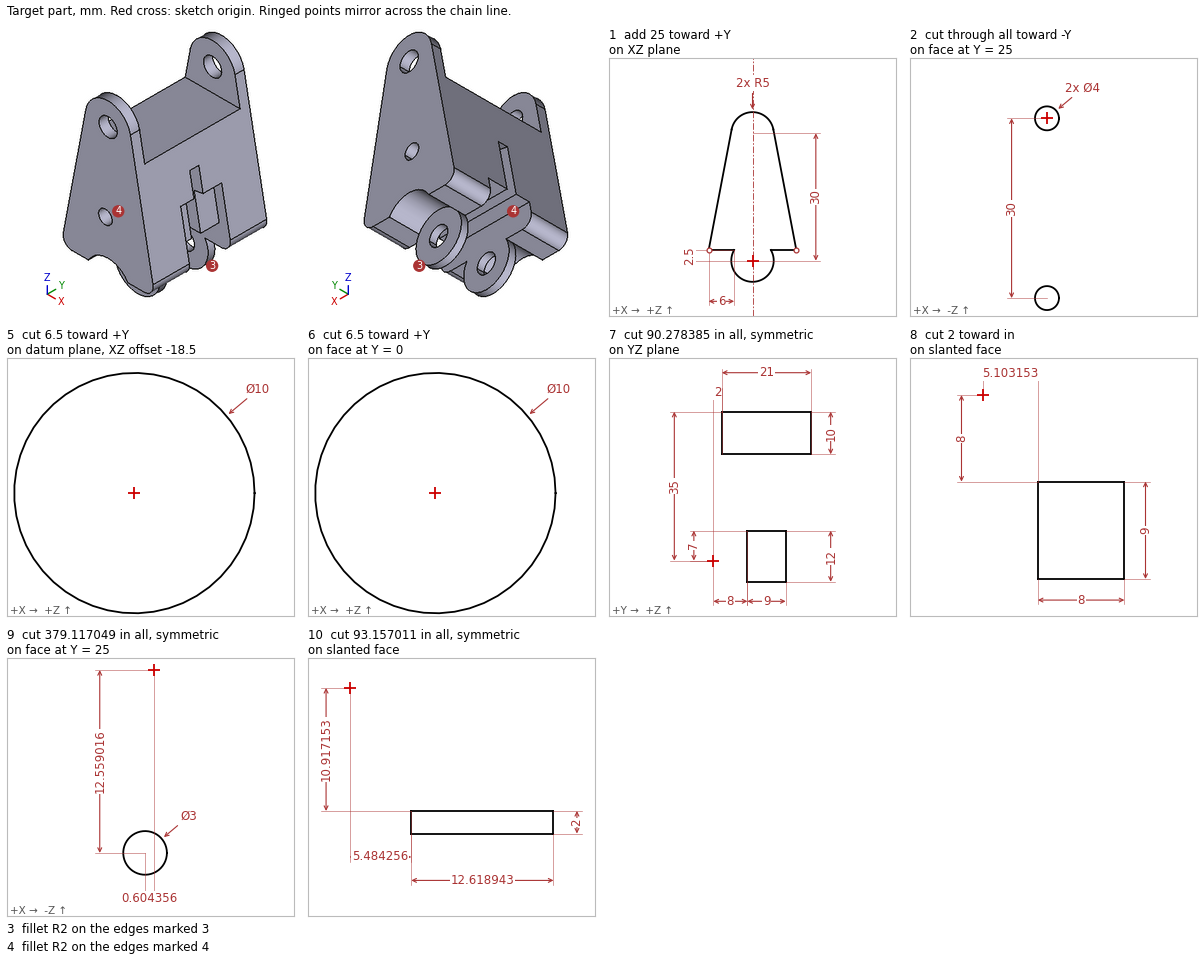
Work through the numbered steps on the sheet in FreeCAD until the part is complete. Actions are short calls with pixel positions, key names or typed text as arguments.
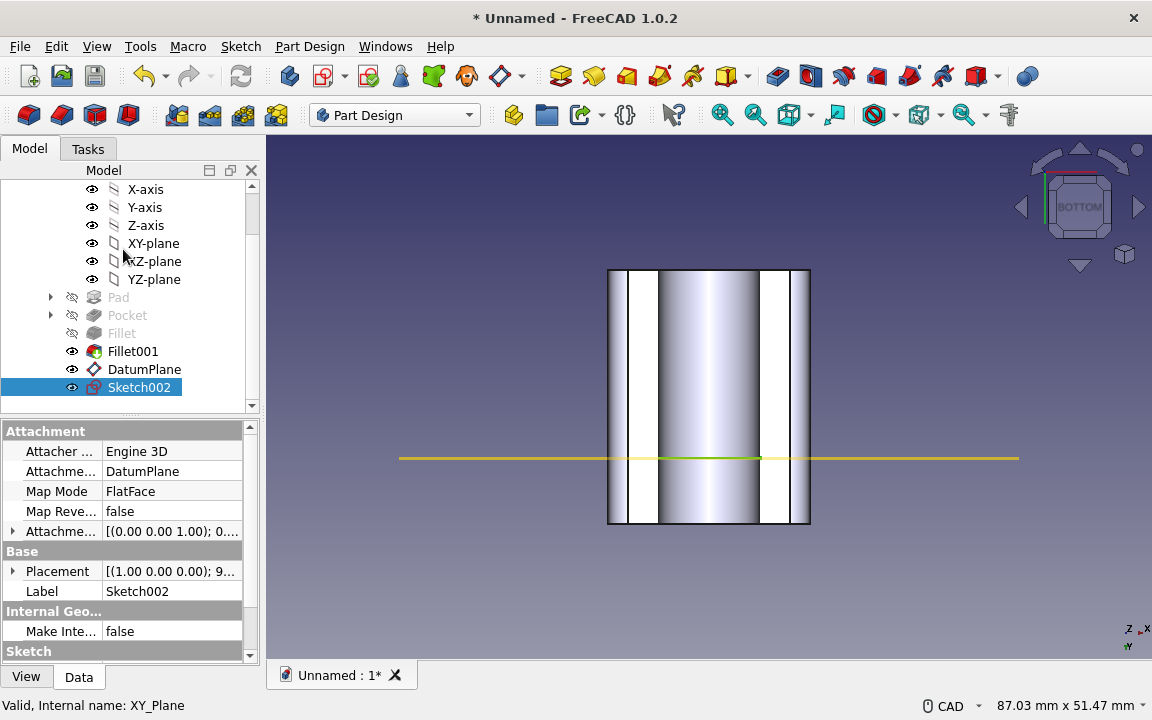
click(778, 76)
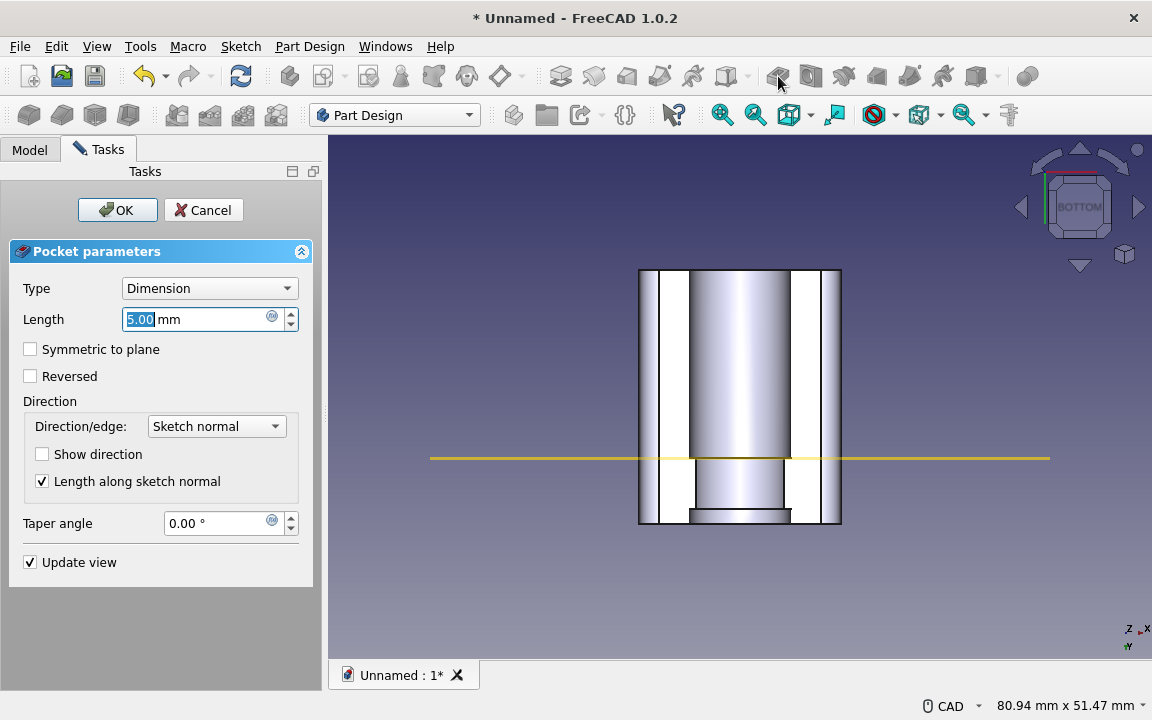
text(6.5)
key(Tab)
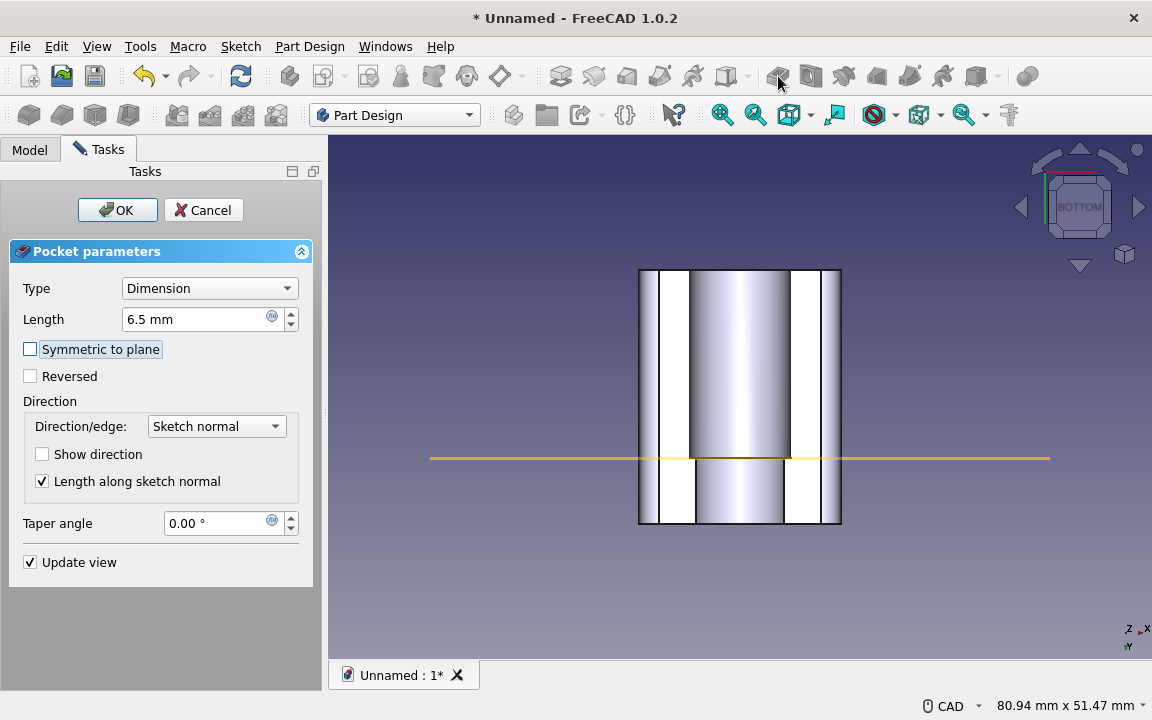
click(118, 210)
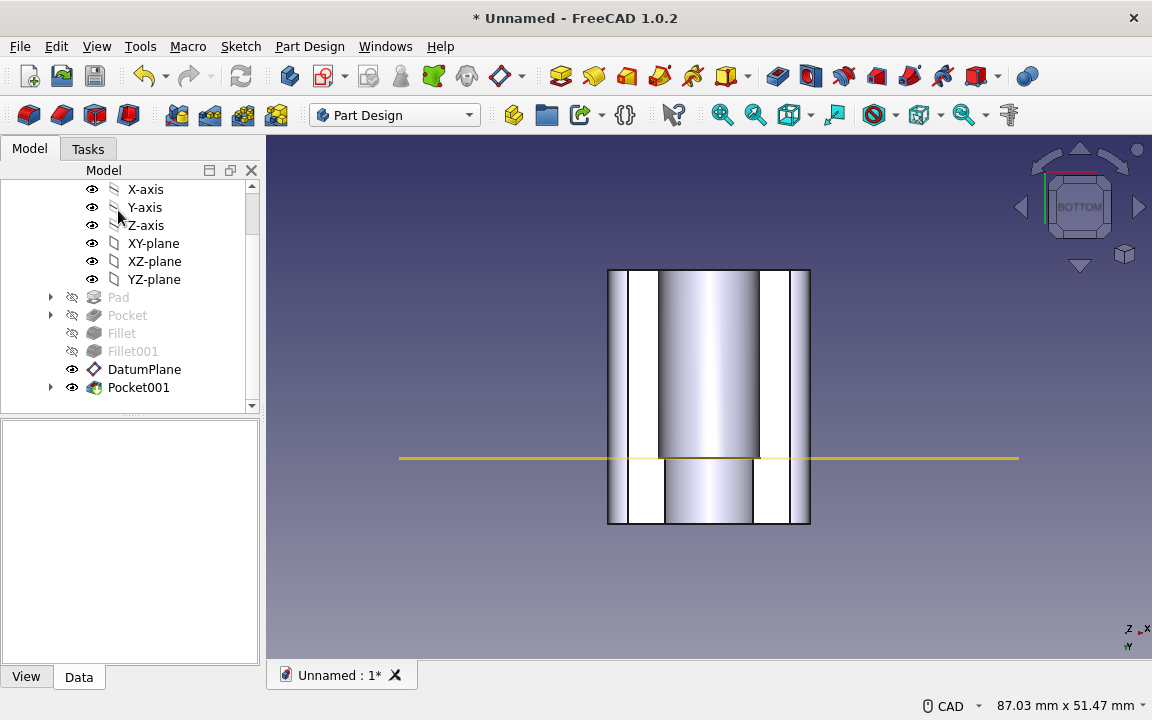
click(117, 369)
key(space)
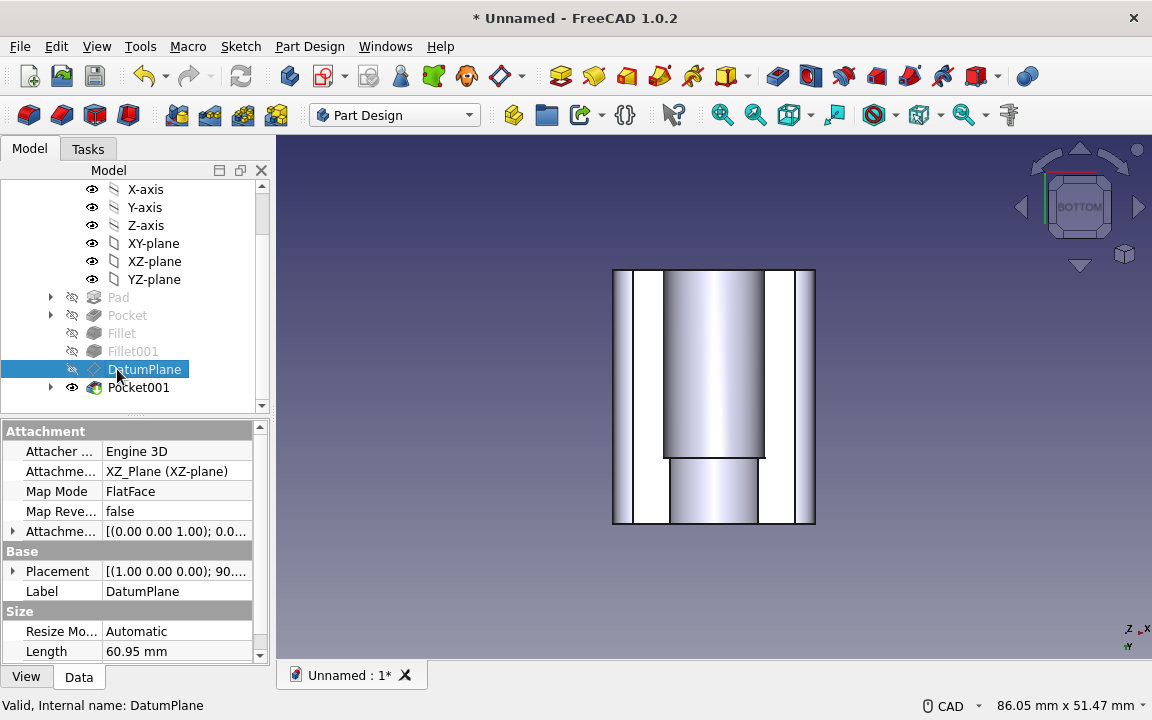
key(0)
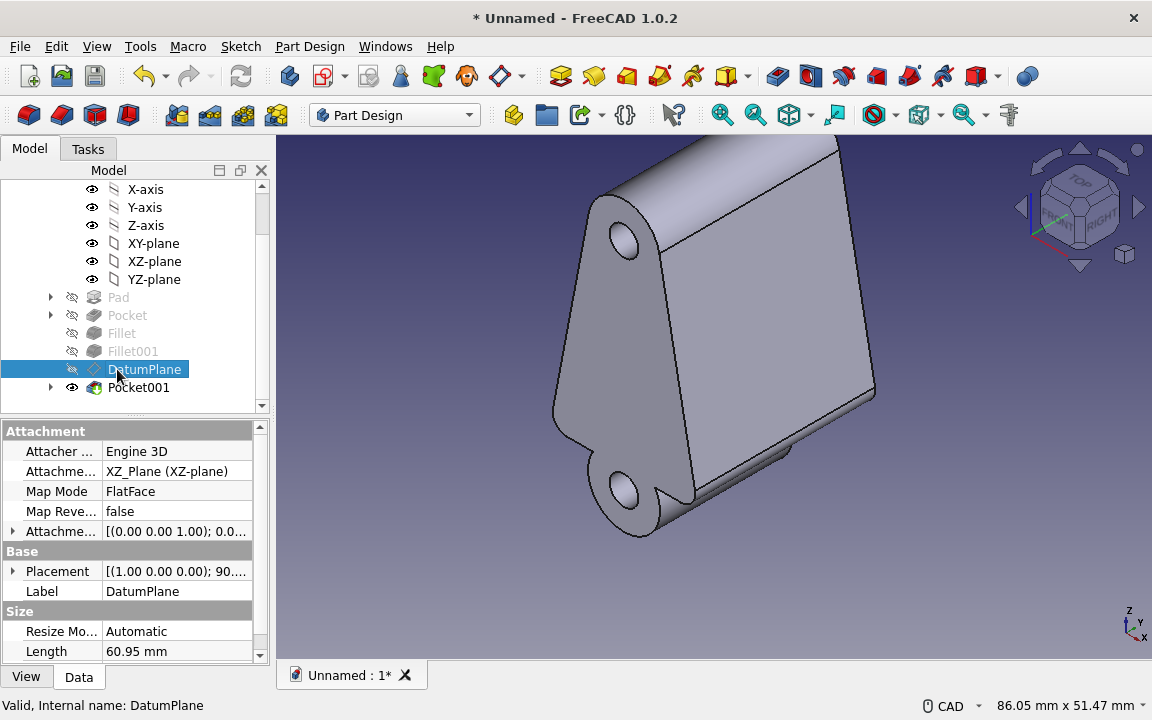
key(v)
key(f)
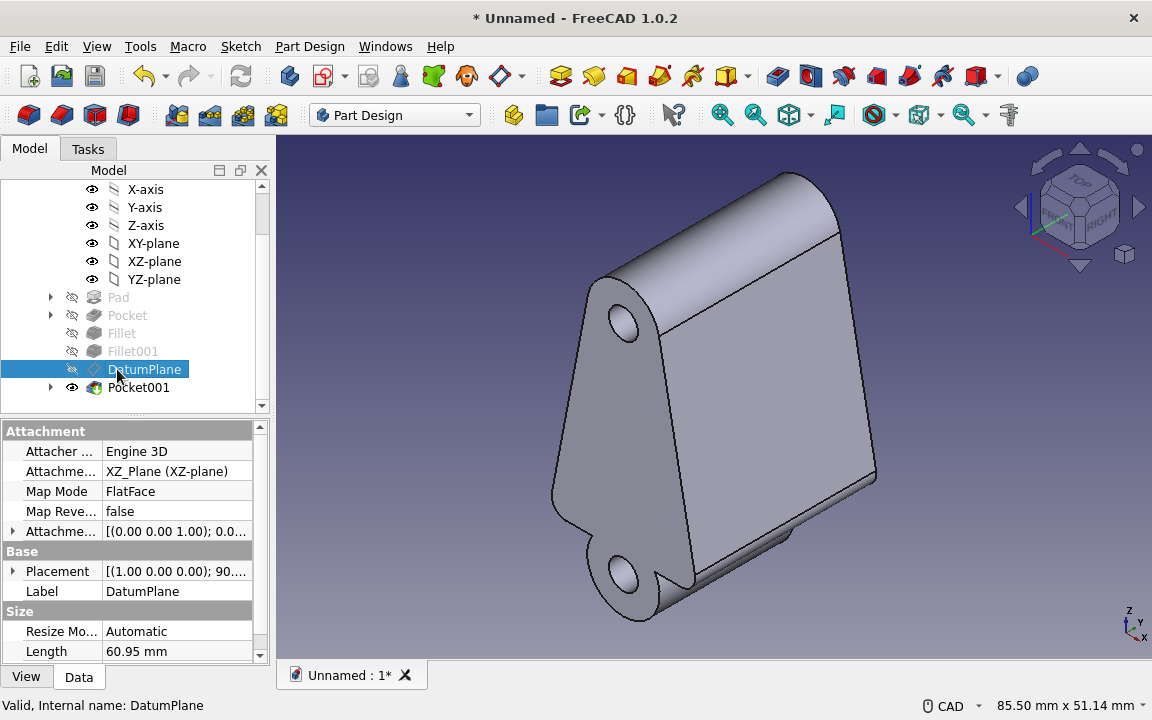
click(623, 448)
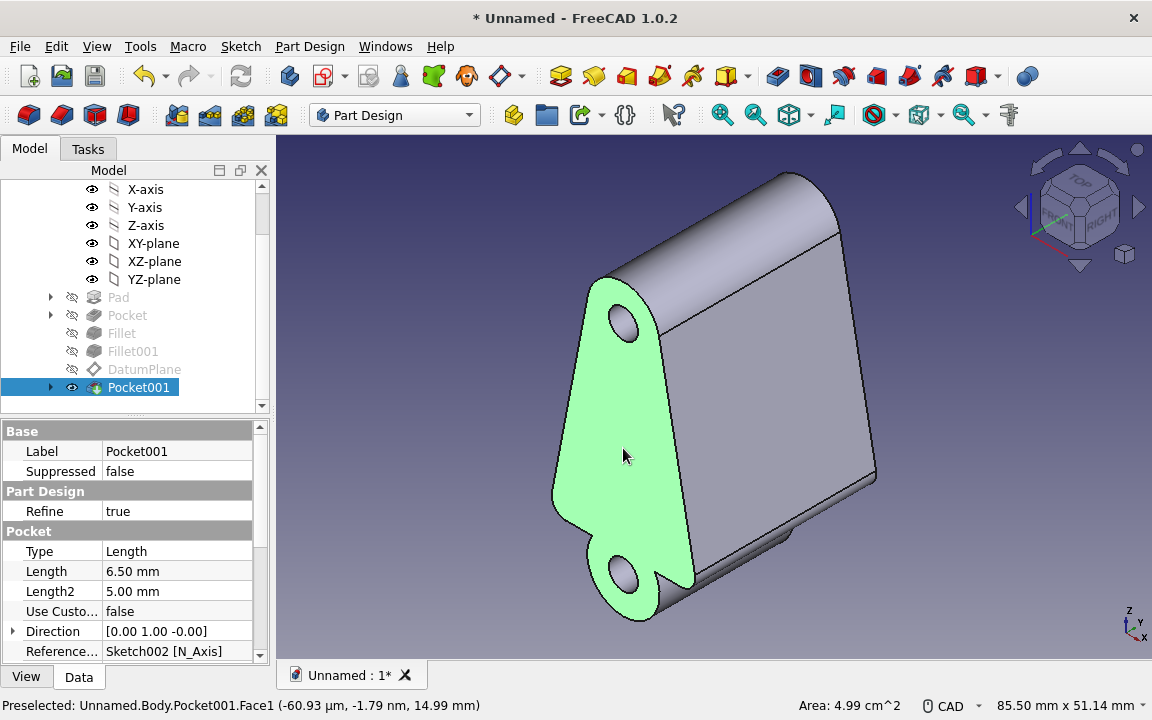
click(322, 76)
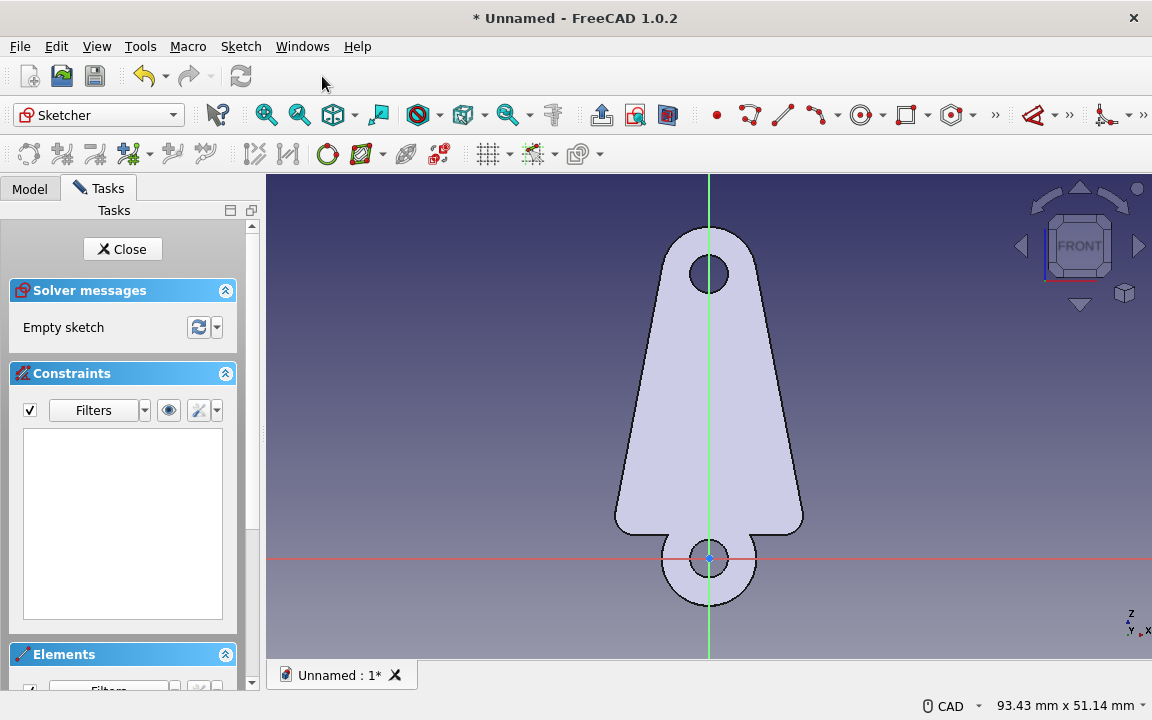
scroll(739, 620, up, 6)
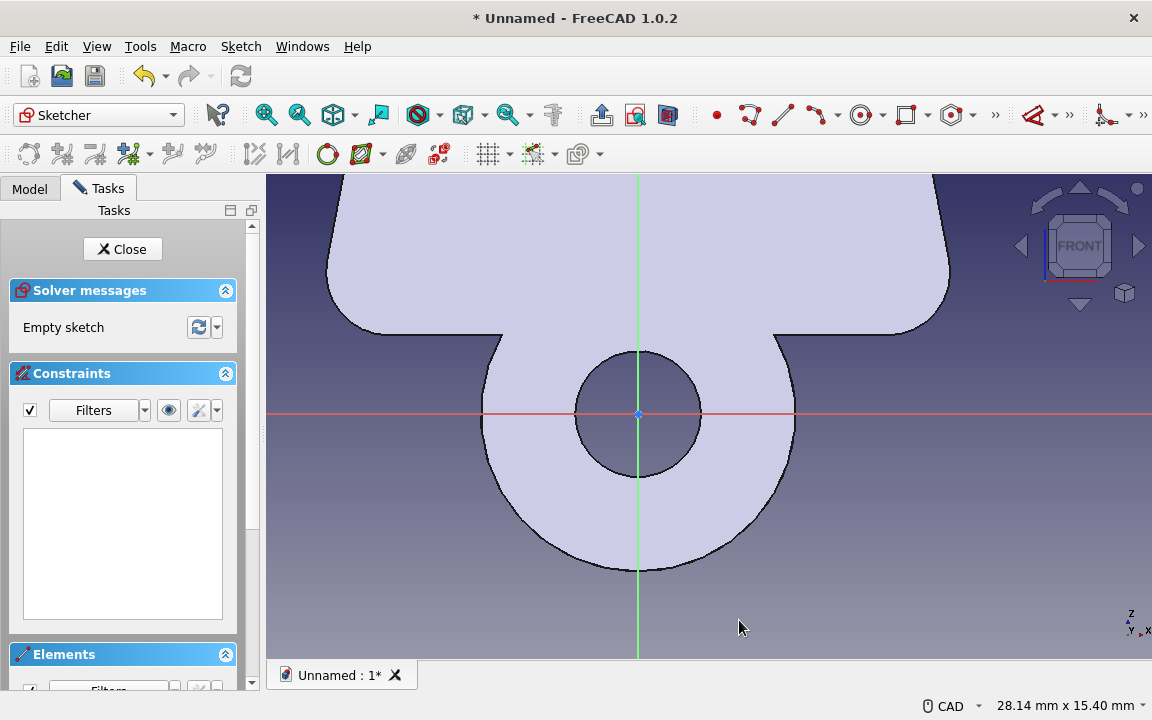
key(g)
key(c)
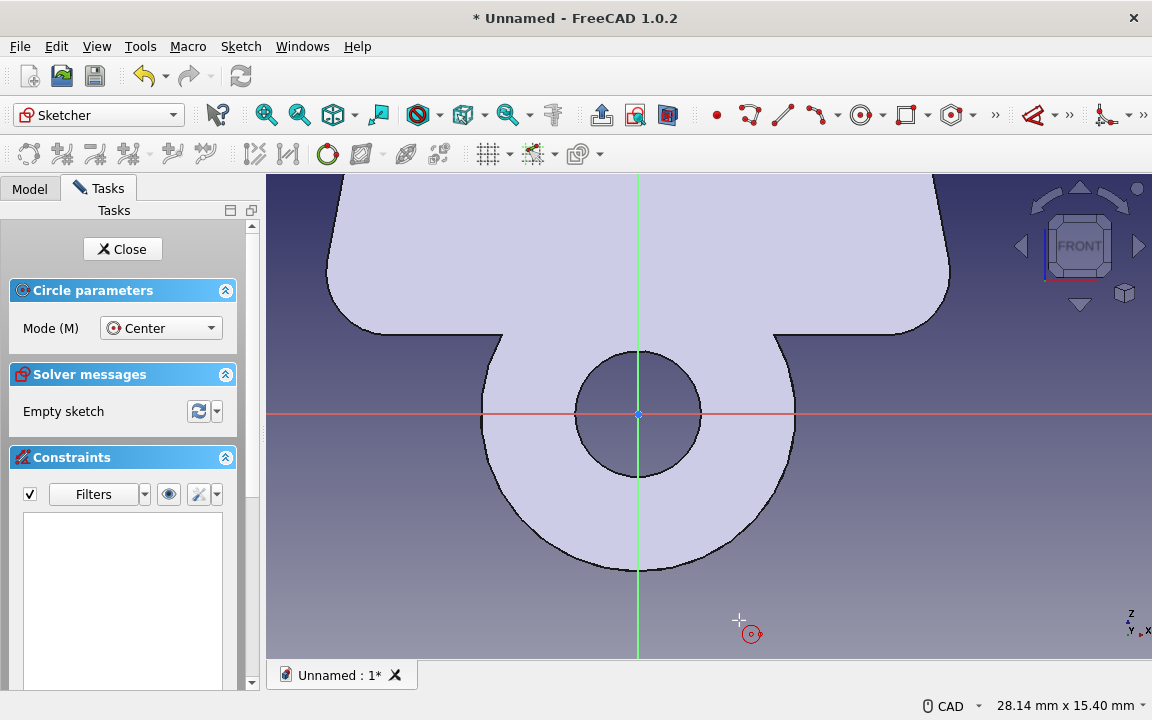
click(638, 414)
move(749, 303)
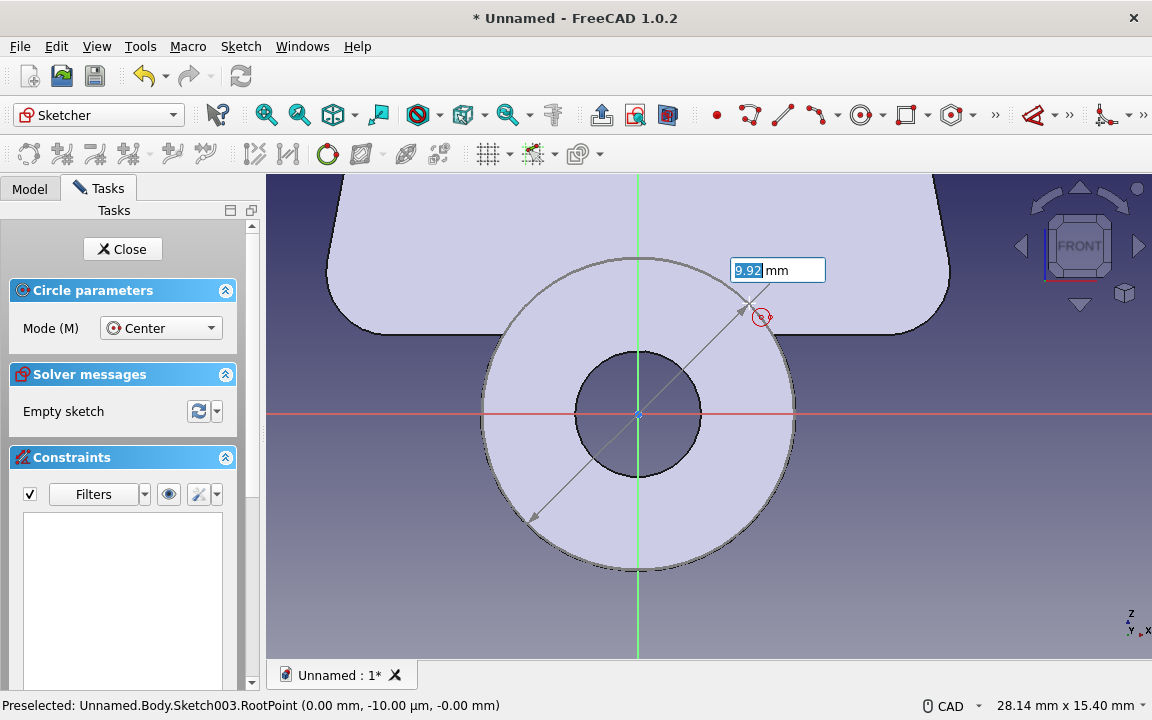
text(10)
key(Return)
key(Escape)